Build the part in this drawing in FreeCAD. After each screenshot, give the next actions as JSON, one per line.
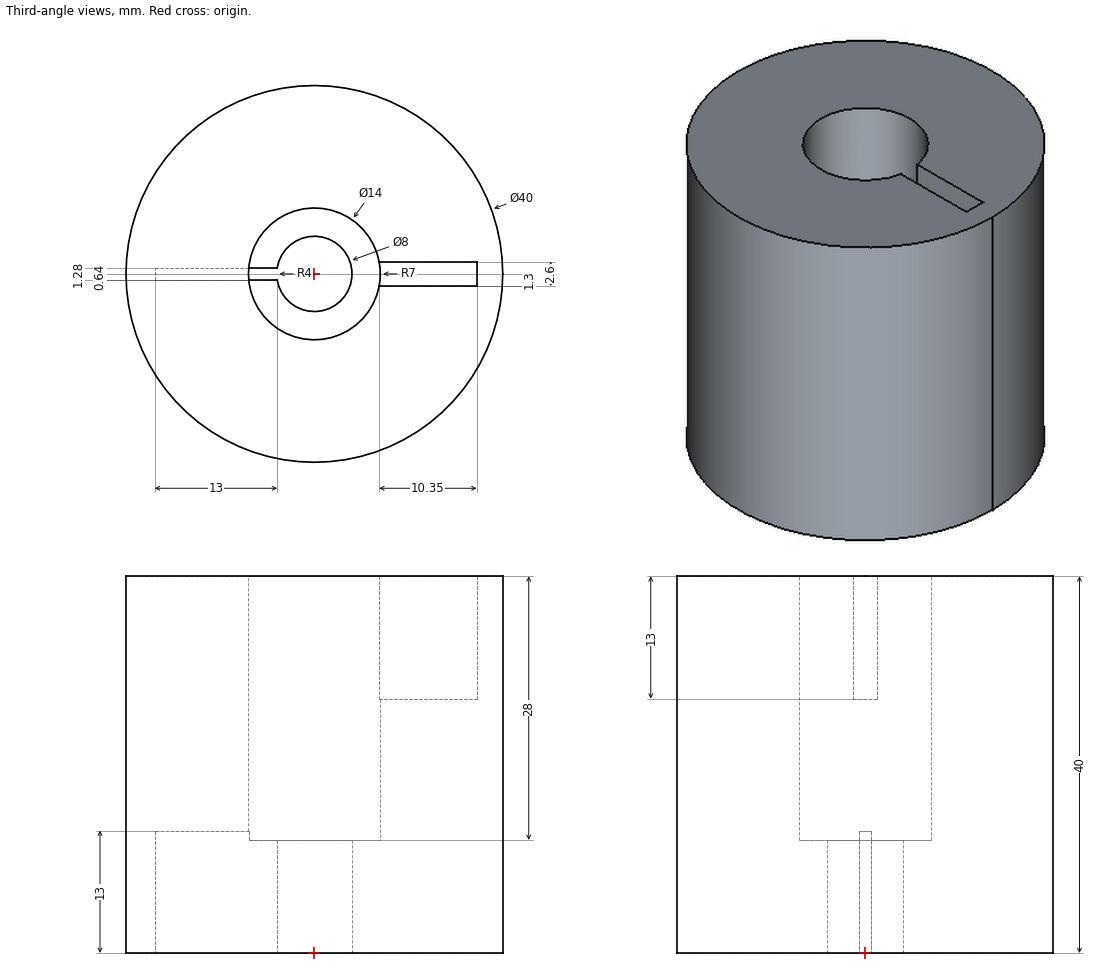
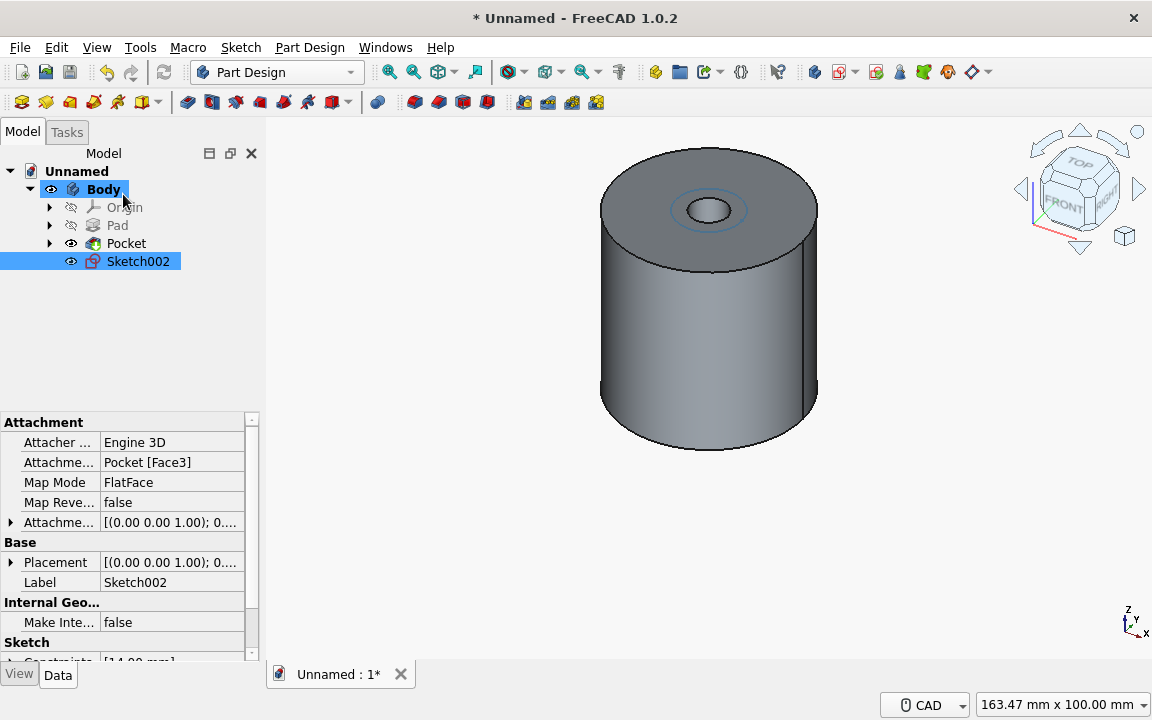
{"action": "left_click", "coordinate": [188, 102]}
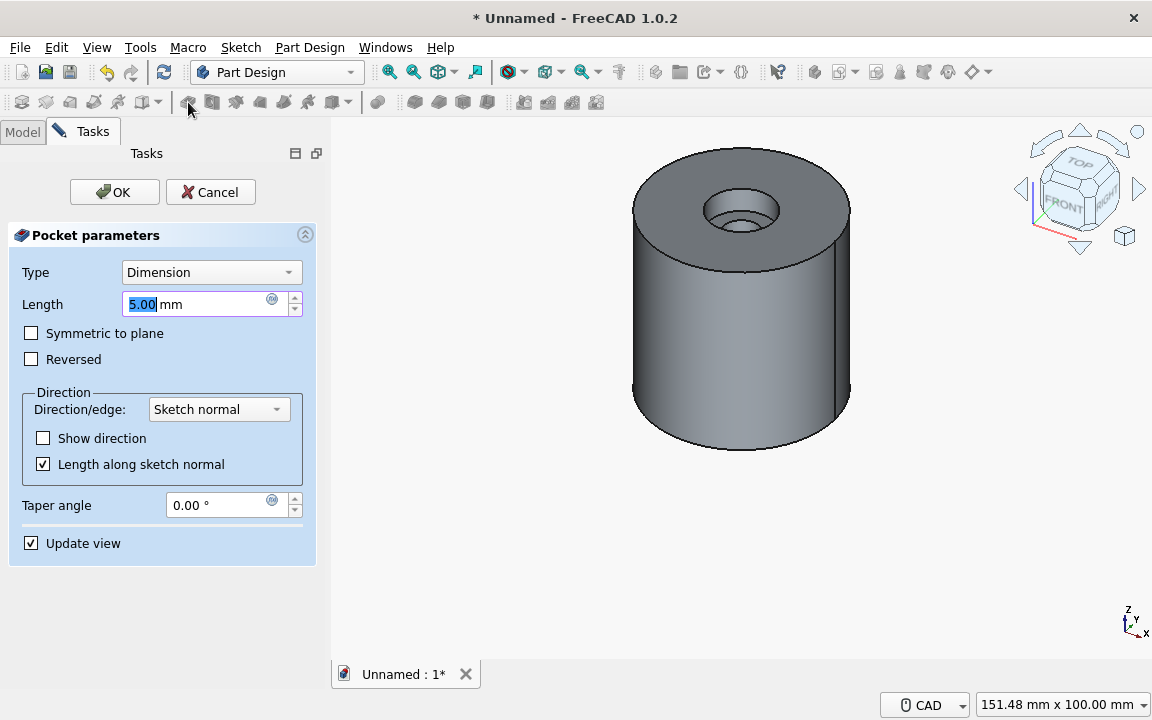
{"action": "type", "text": "28"}
{"action": "key", "text": "Tab"}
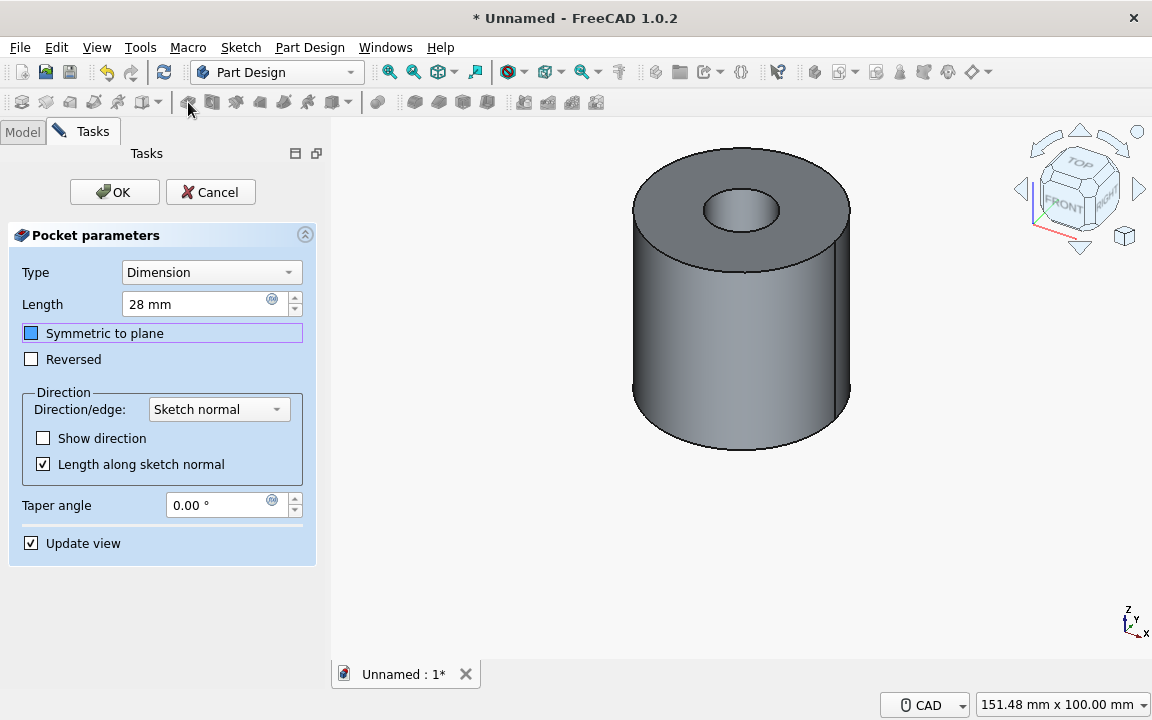
{"action": "left_click", "coordinate": [115, 192]}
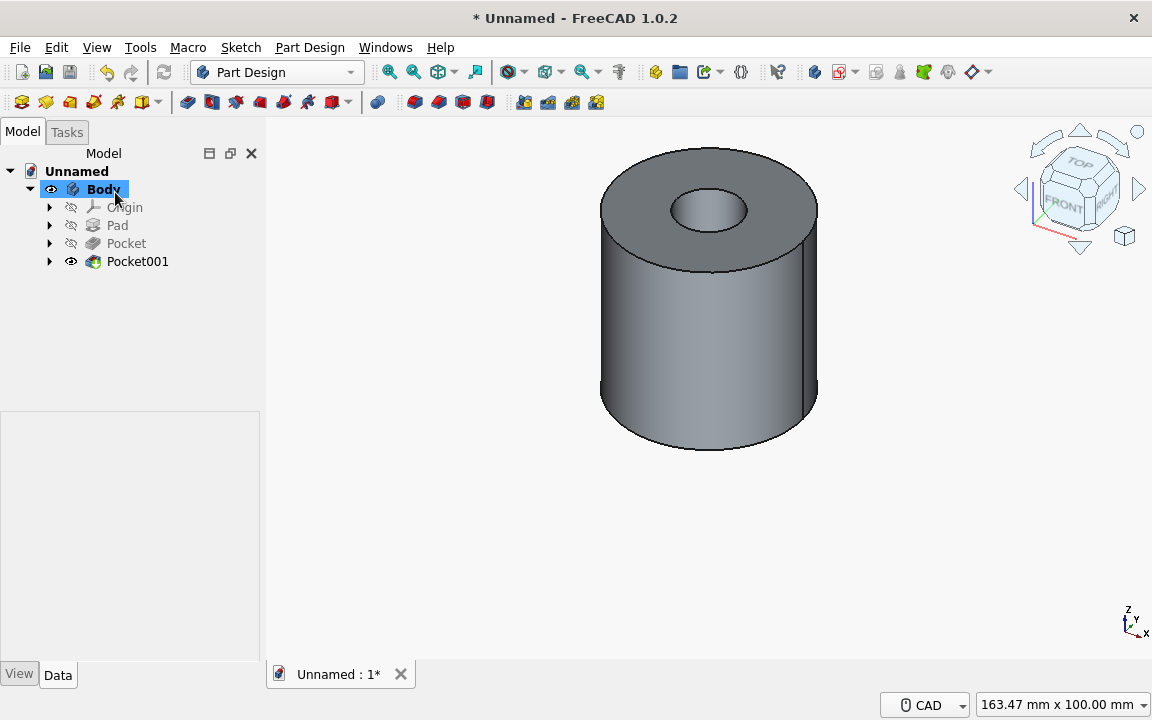
{"action": "left_click", "coordinate": [671, 176]}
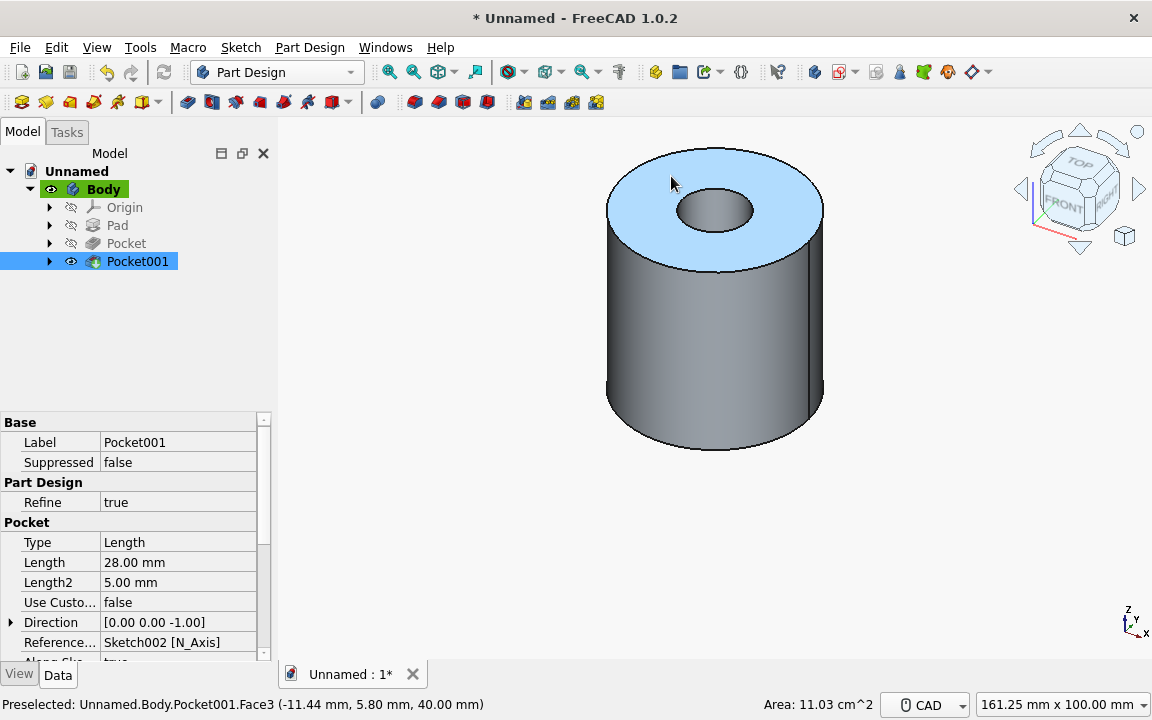
{"action": "left_click", "coordinate": [840, 72]}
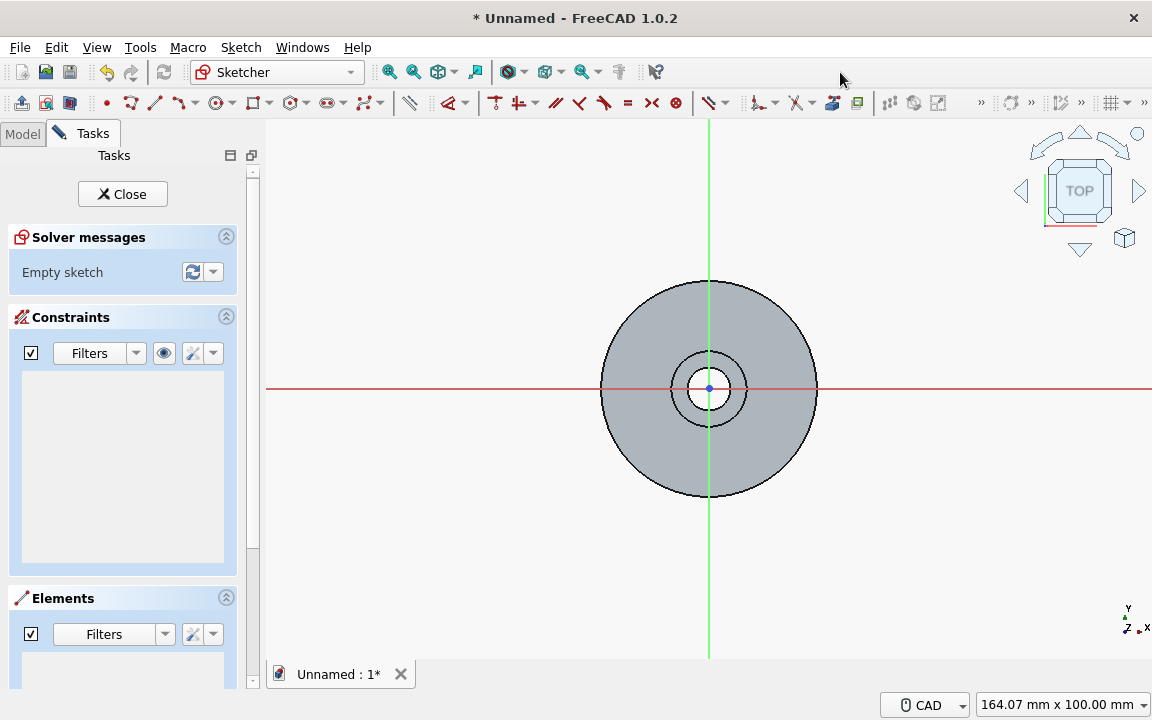
{"action": "scroll", "coordinate": [785, 389], "scroll_direction": "up", "scroll_amount": 8}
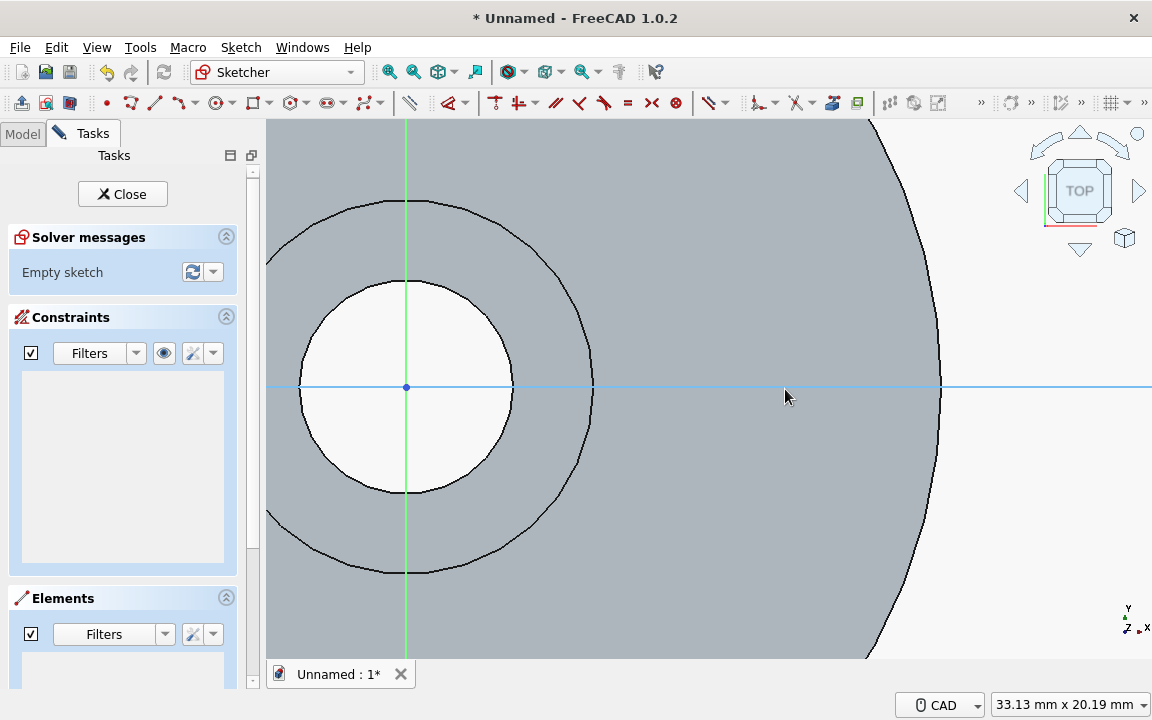
{"action": "key", "text": "g m"}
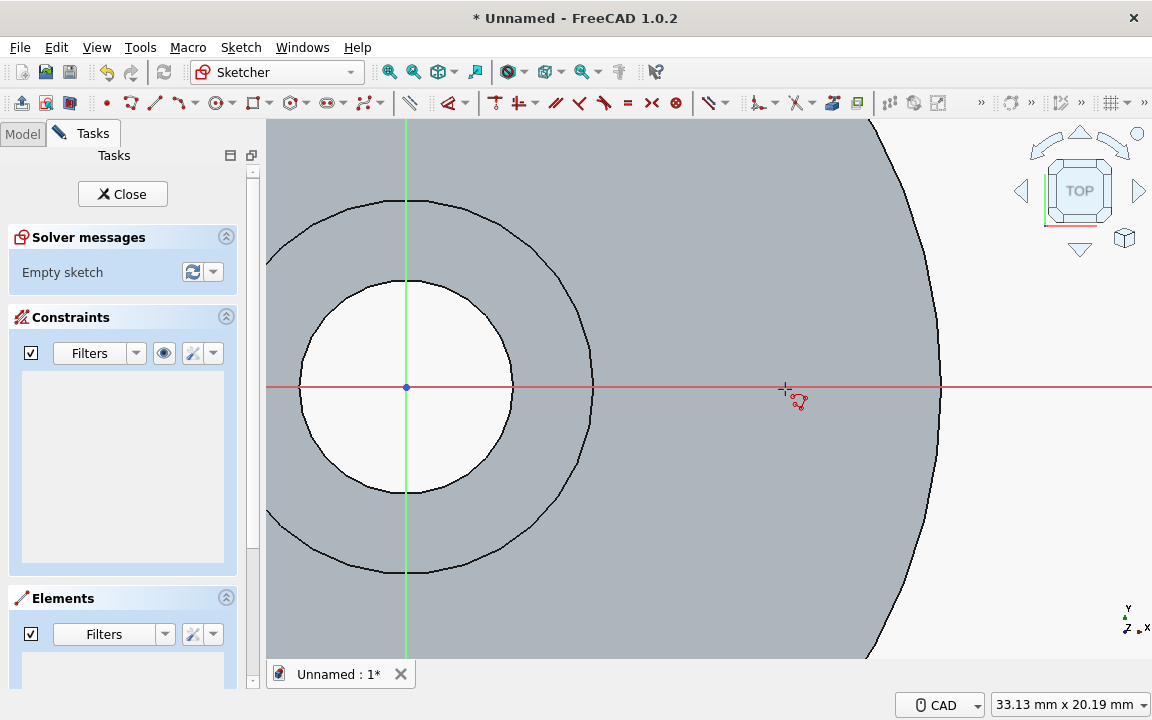
{"action": "left_click", "coordinate": [590, 422]}
{"action": "left_click", "coordinate": [867, 422]}
{"action": "left_click", "coordinate": [867, 352]}
{"action": "left_click", "coordinate": [590, 352]}
{"action": "right_click", "coordinate": [590, 352]}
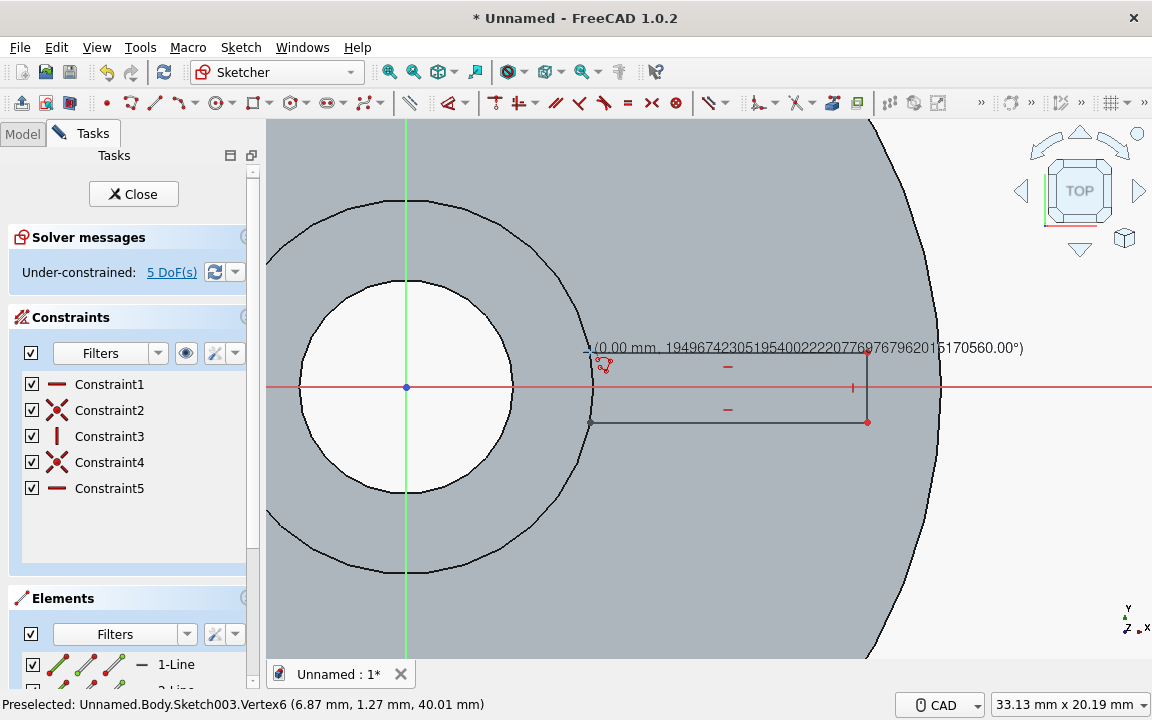
{"action": "left_click", "coordinate": [180, 104]}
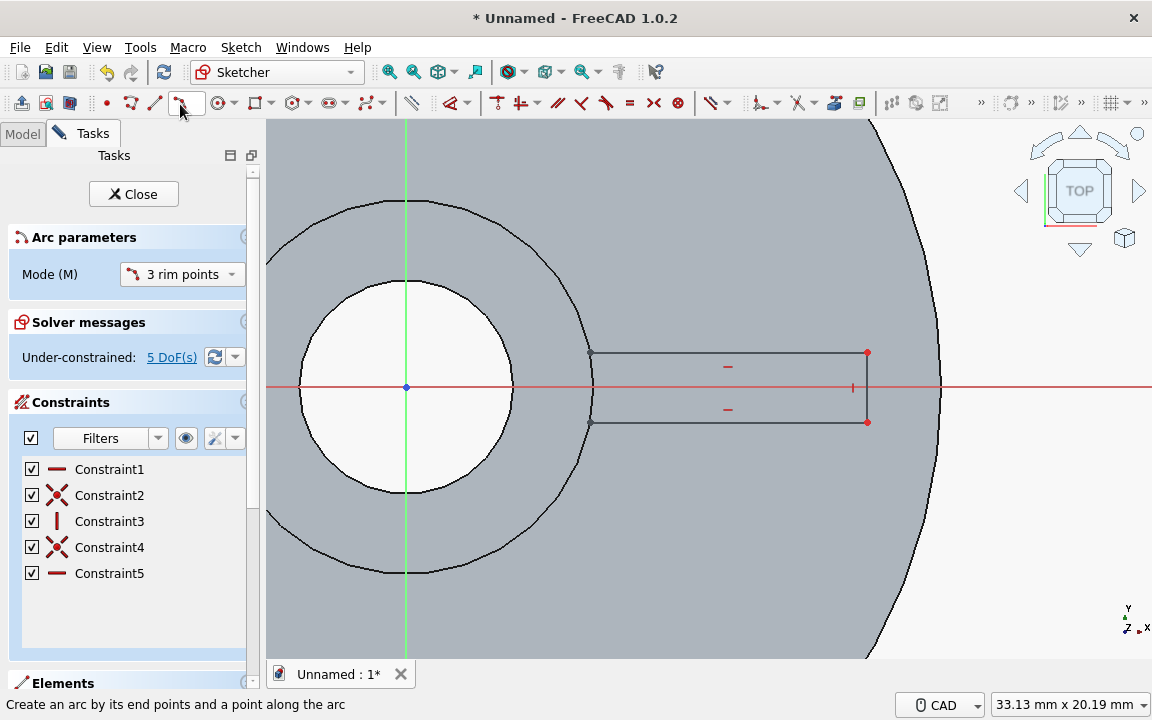
{"action": "left_click", "coordinate": [590, 353]}
{"action": "left_click", "coordinate": [590, 423]}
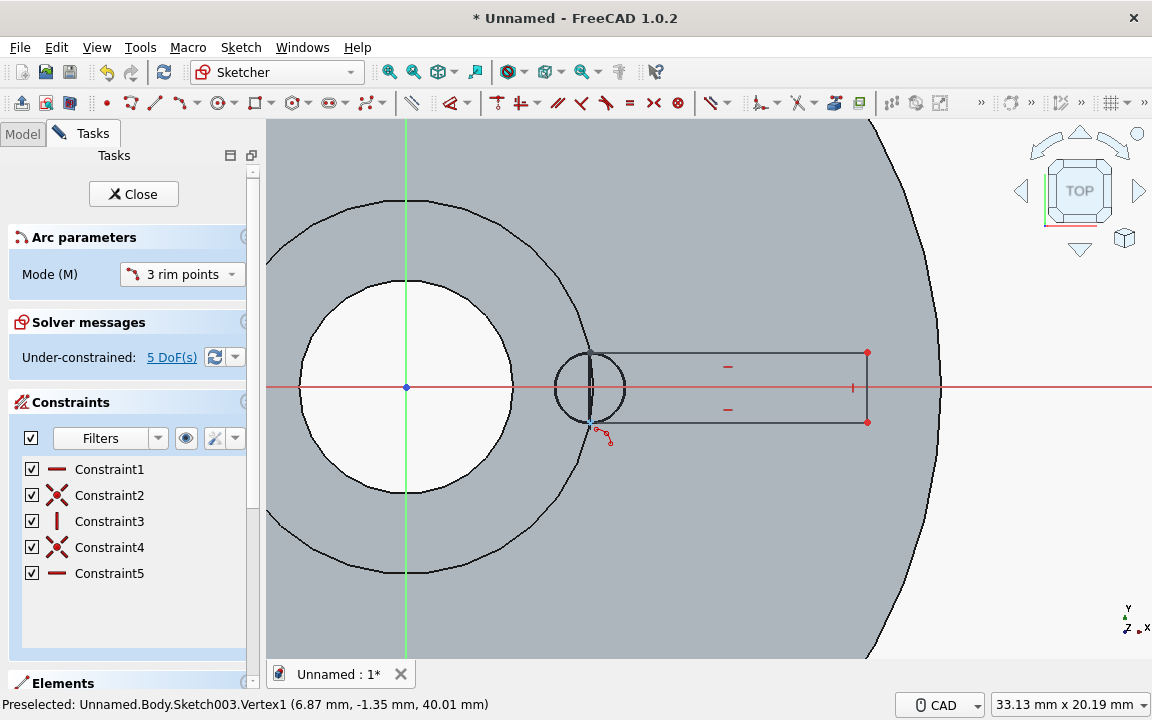
{"action": "scroll", "coordinate": [593, 394], "scroll_direction": "up", "scroll_amount": 9}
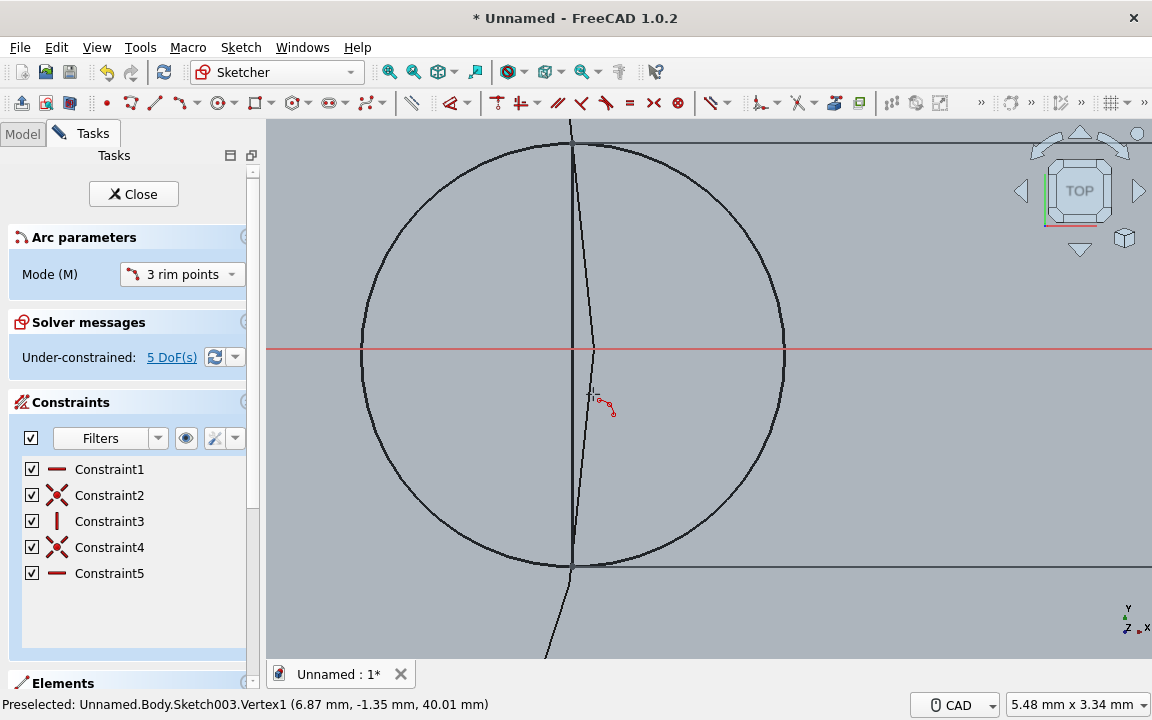
{"action": "left_click", "coordinate": [593, 392]}
{"action": "key", "text": "Escape"}